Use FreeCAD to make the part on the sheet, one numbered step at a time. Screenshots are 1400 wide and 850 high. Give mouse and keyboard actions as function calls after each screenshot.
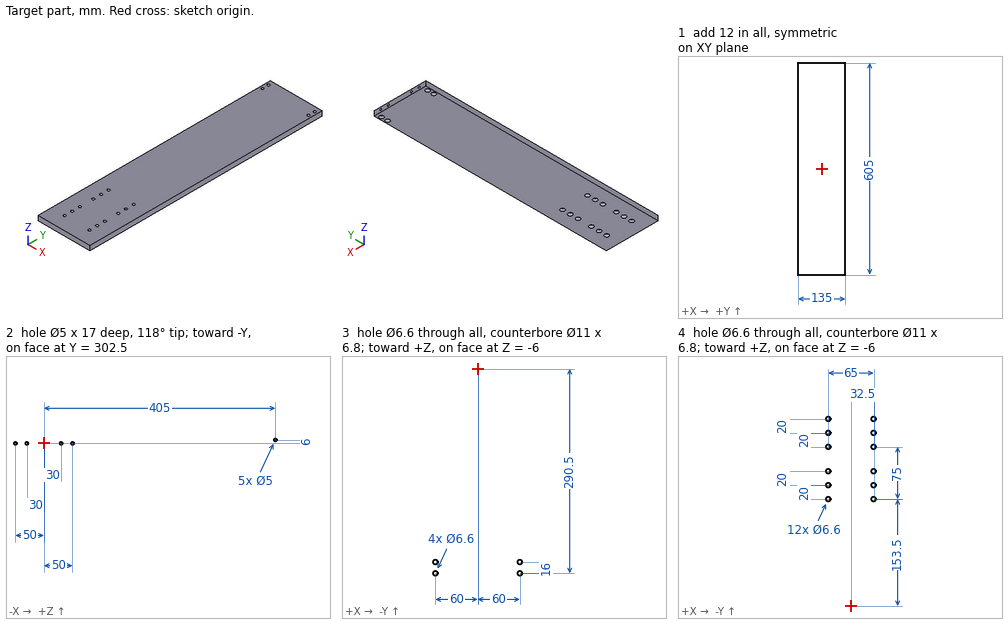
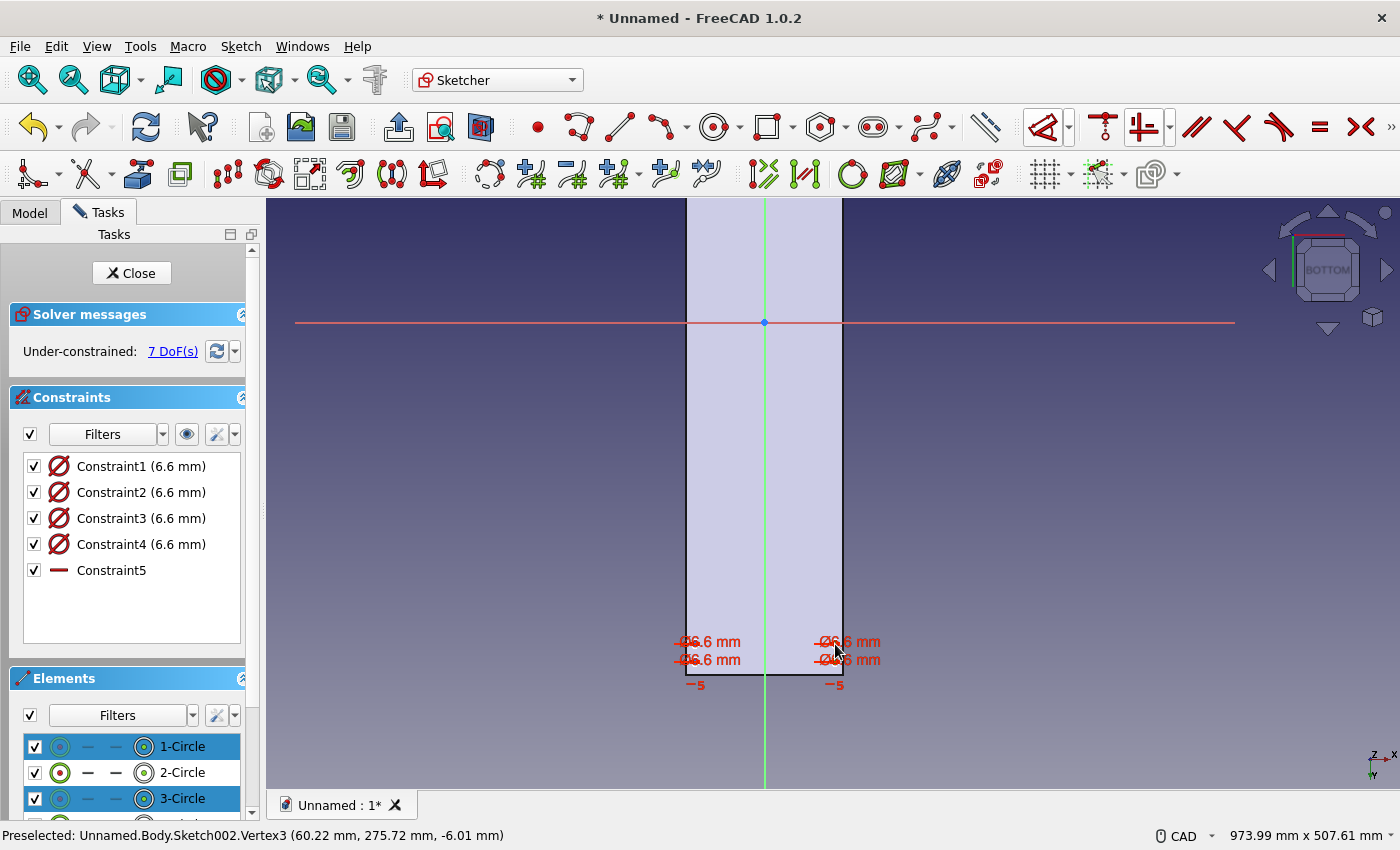
click(1170, 128)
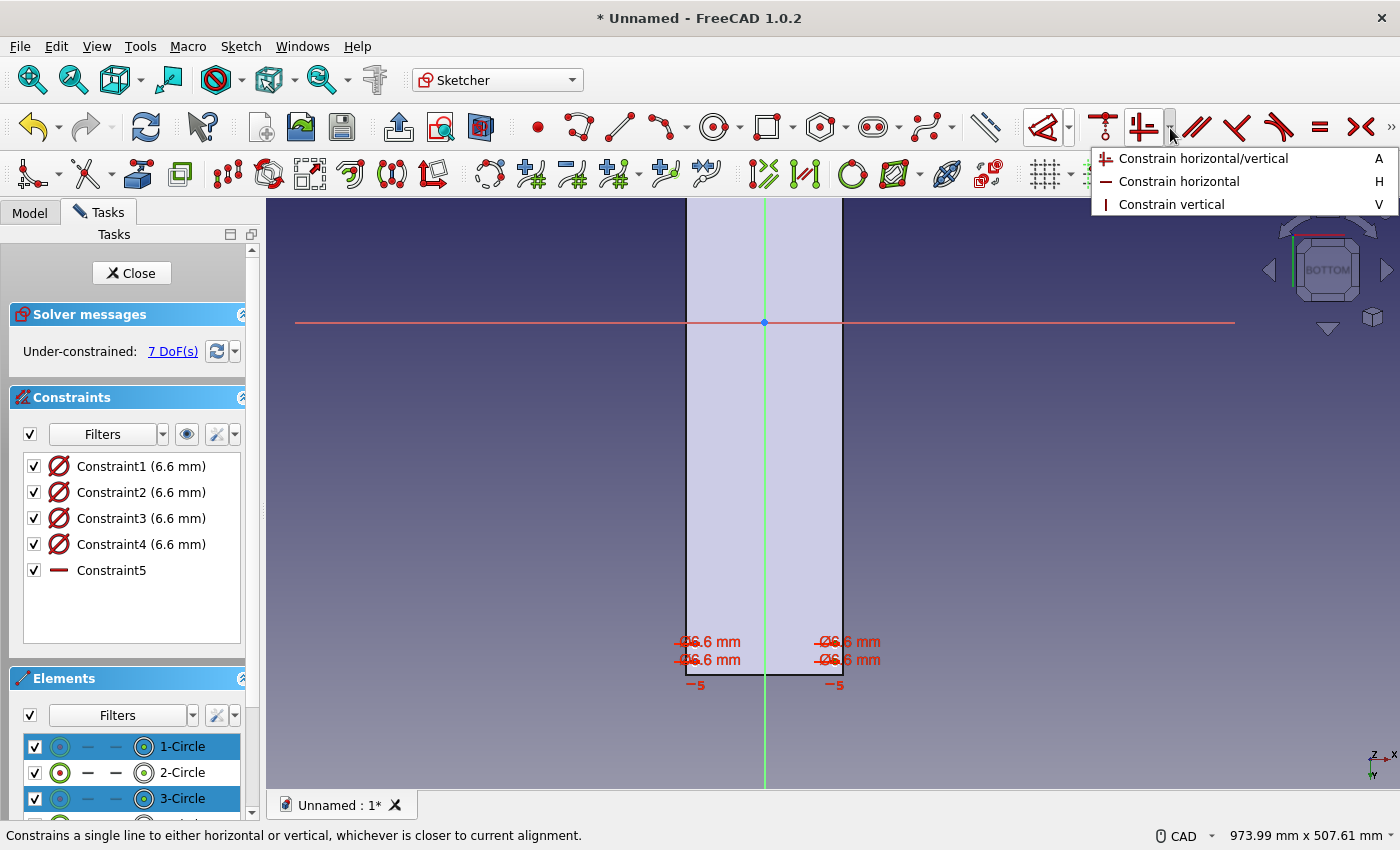
click(1245, 204)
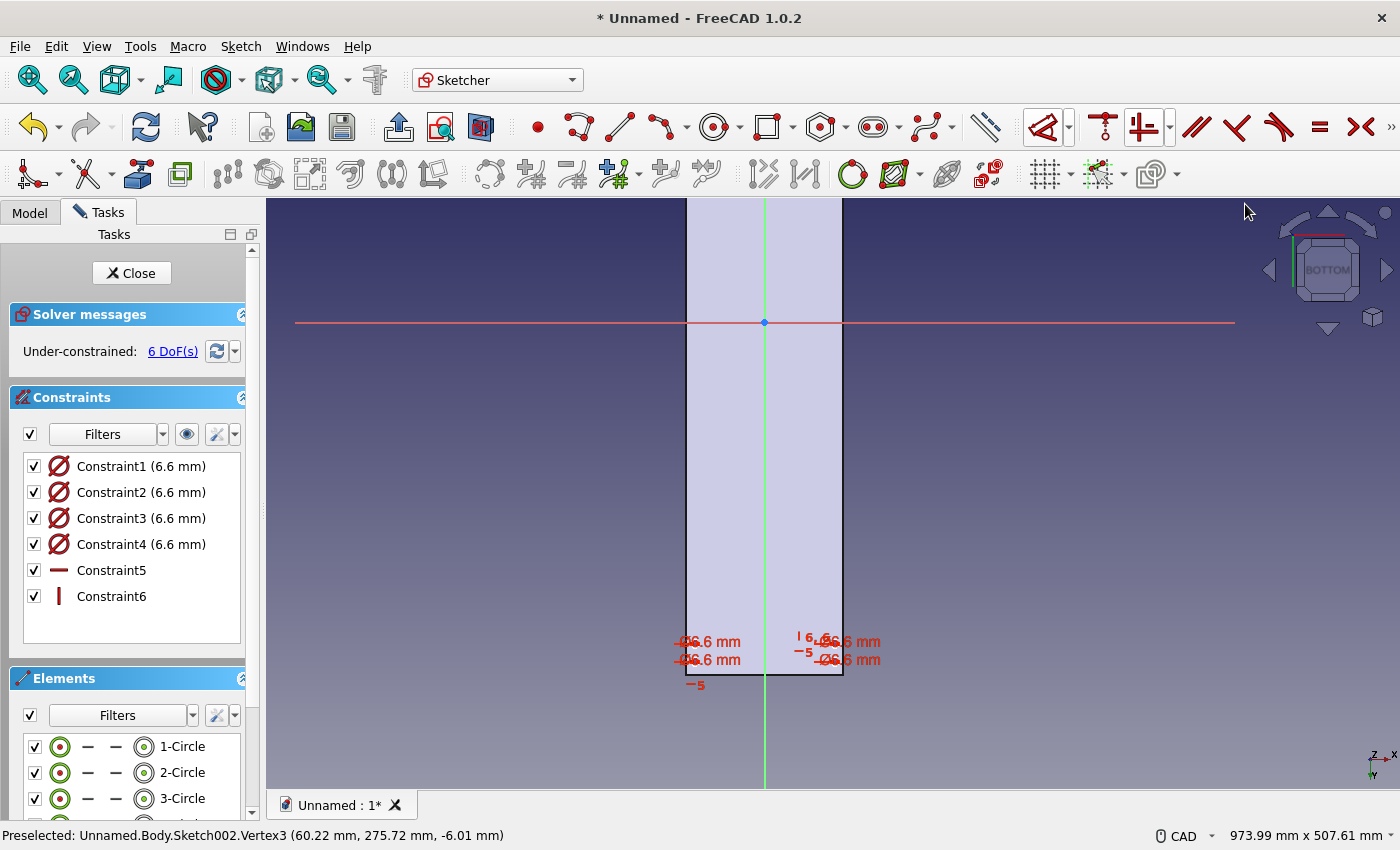
click(695, 662)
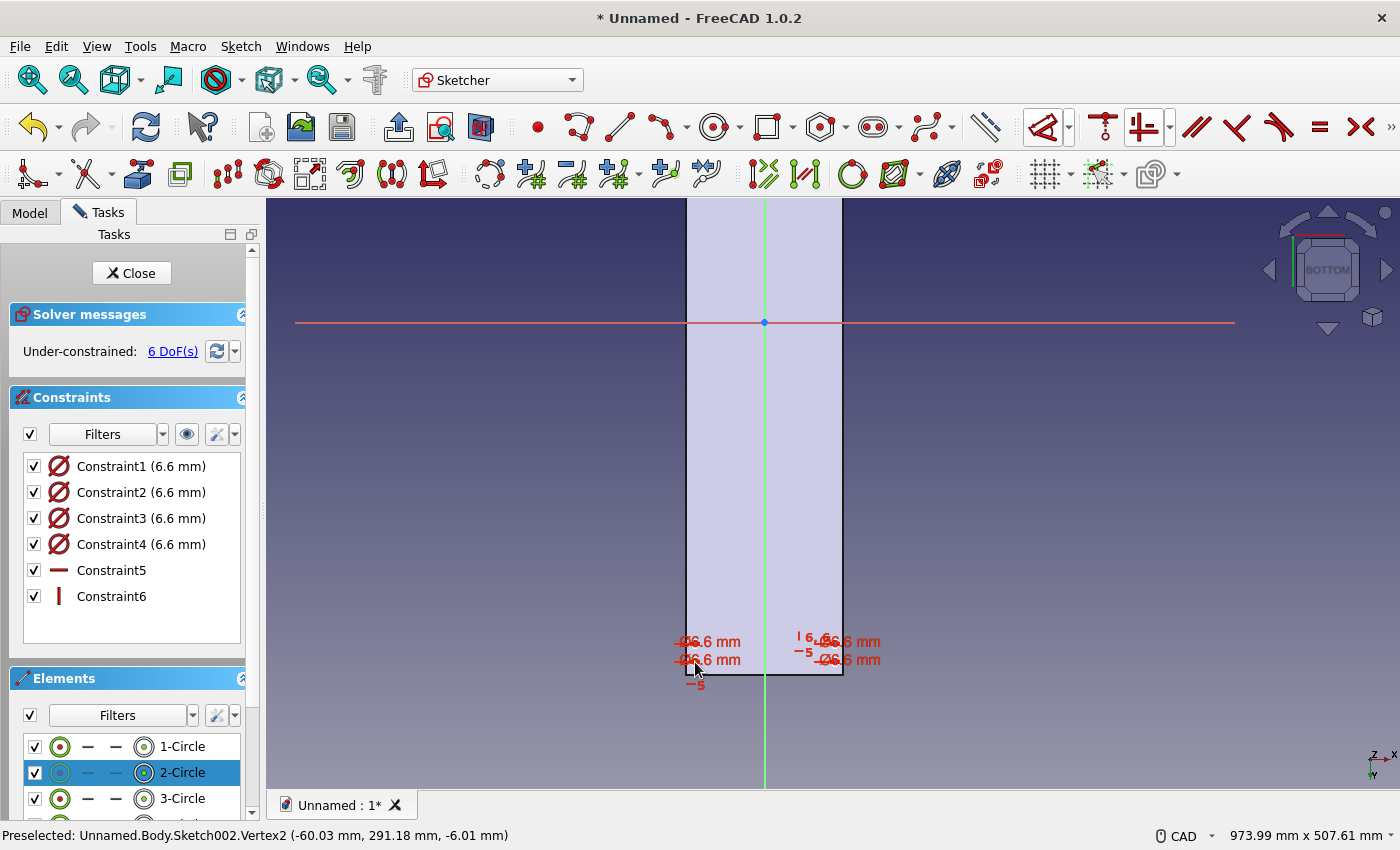
click(695, 644)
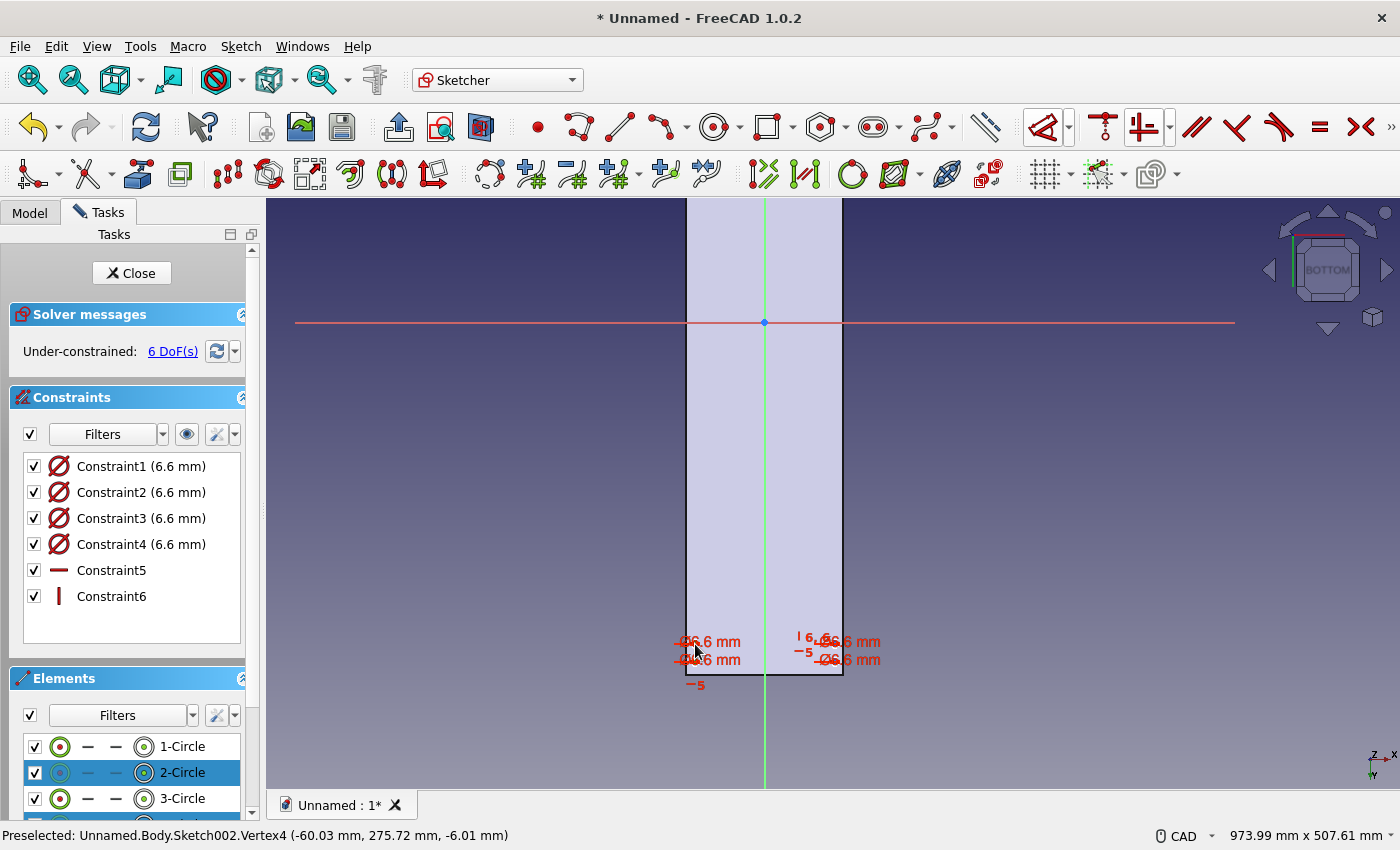
key(v)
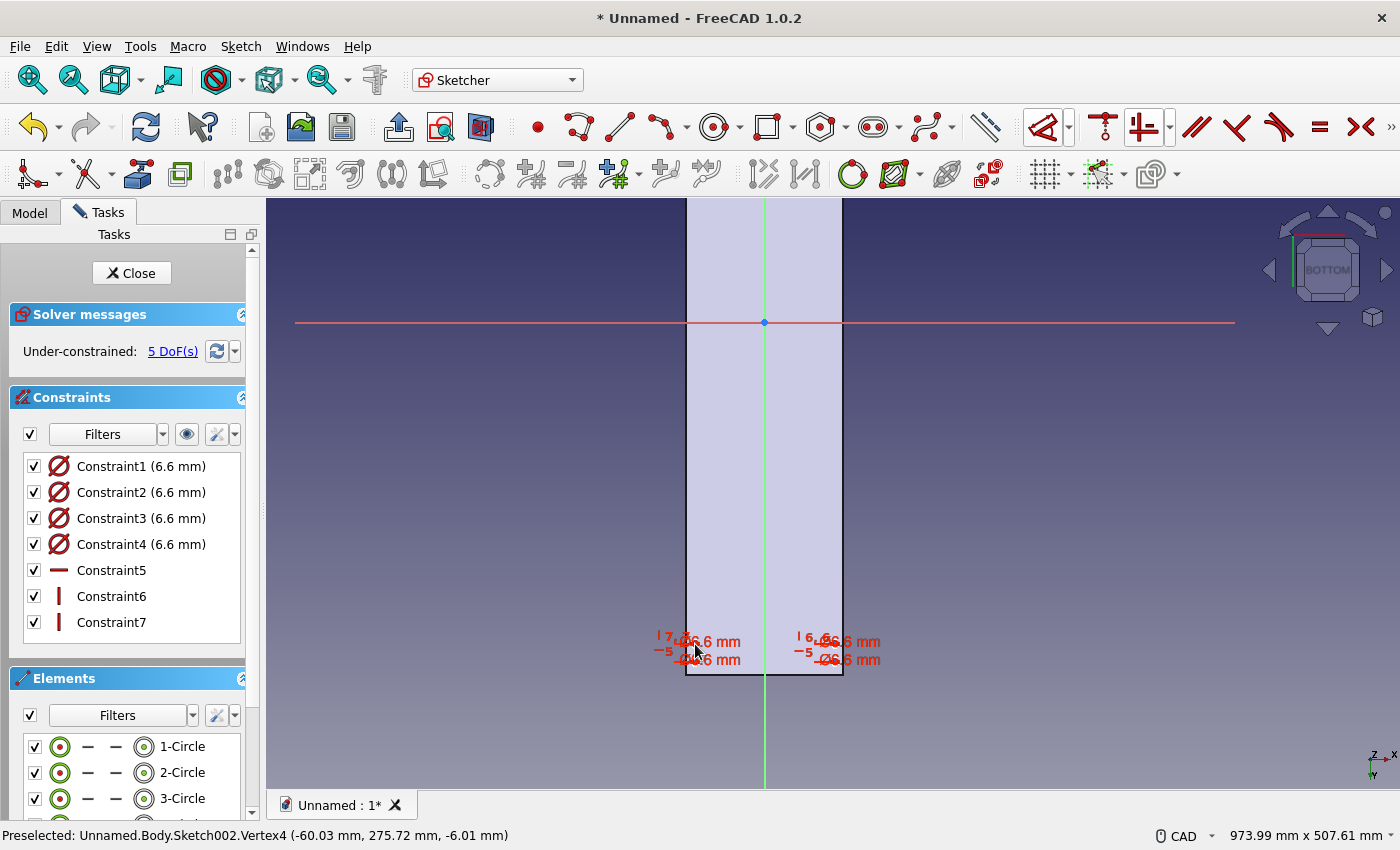
click(835, 644)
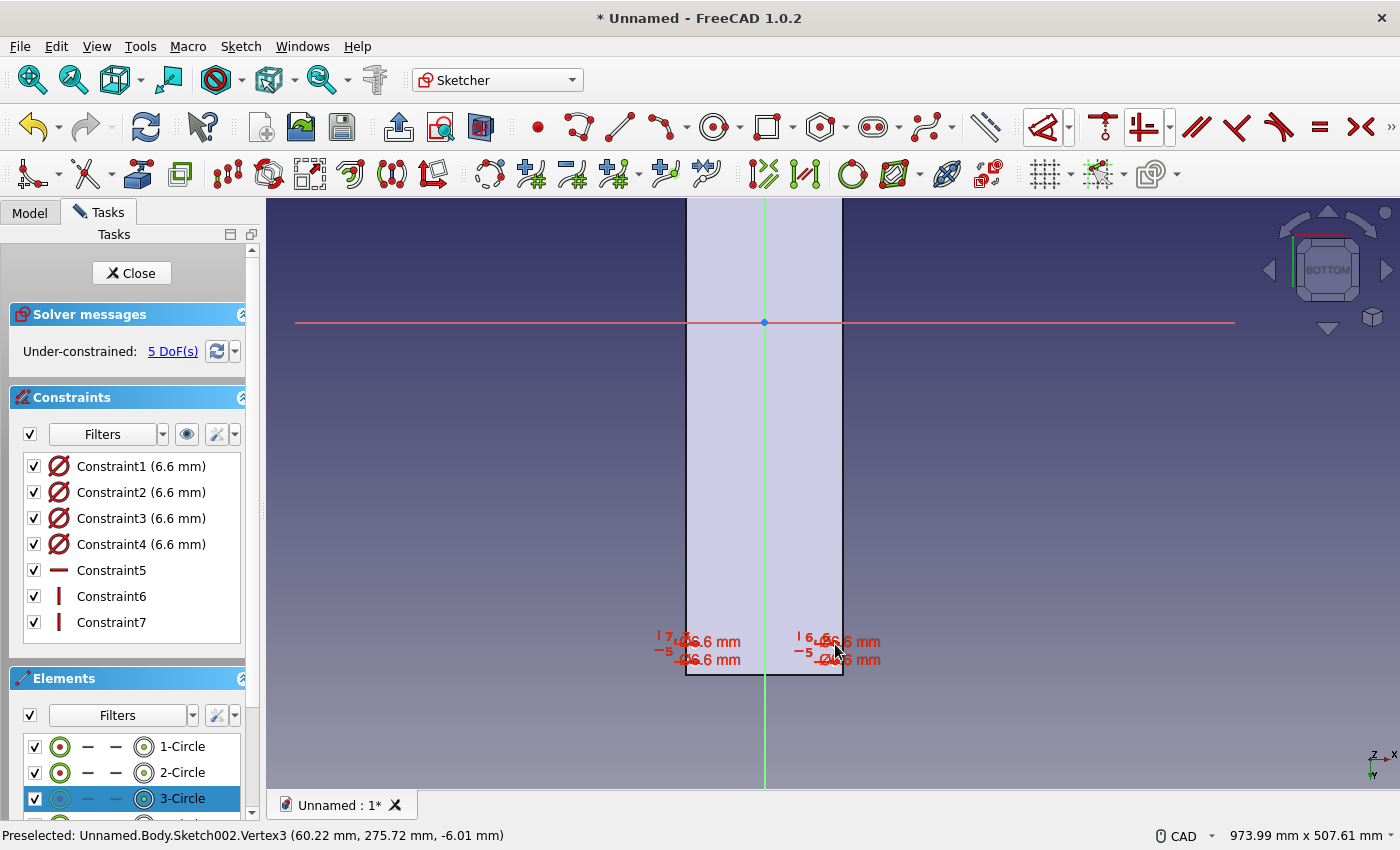
click(695, 644)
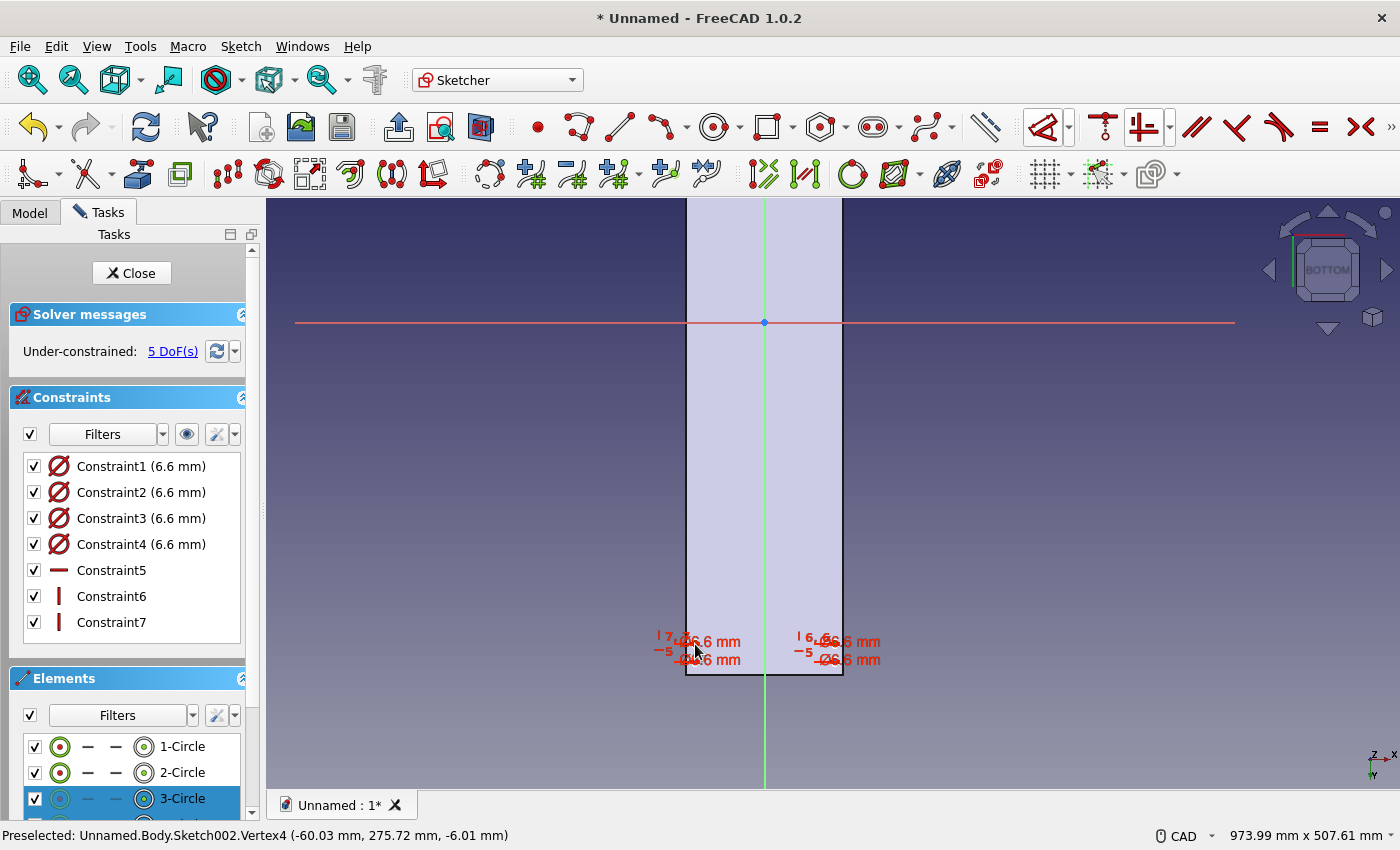
click(1170, 128)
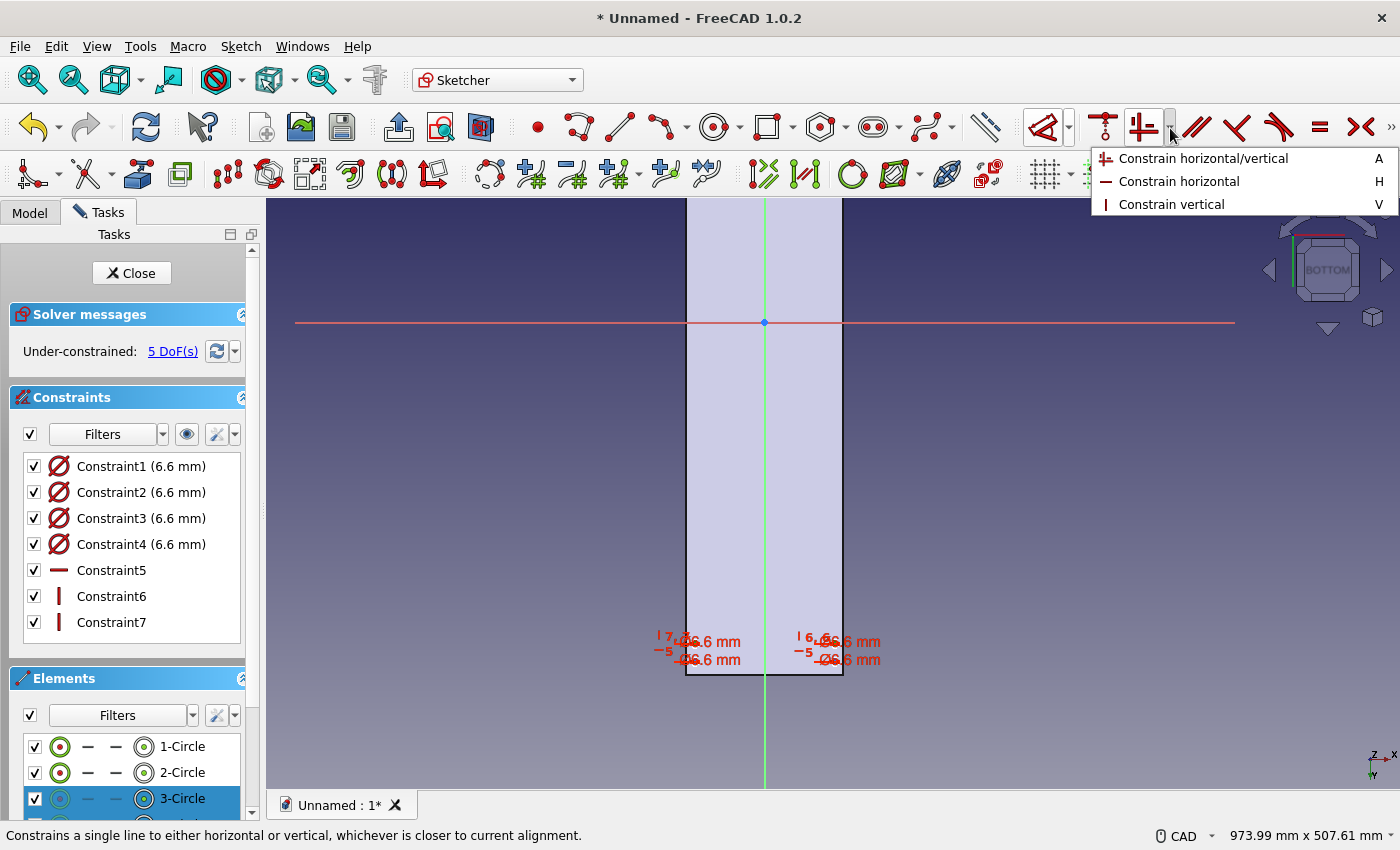
click(1245, 182)